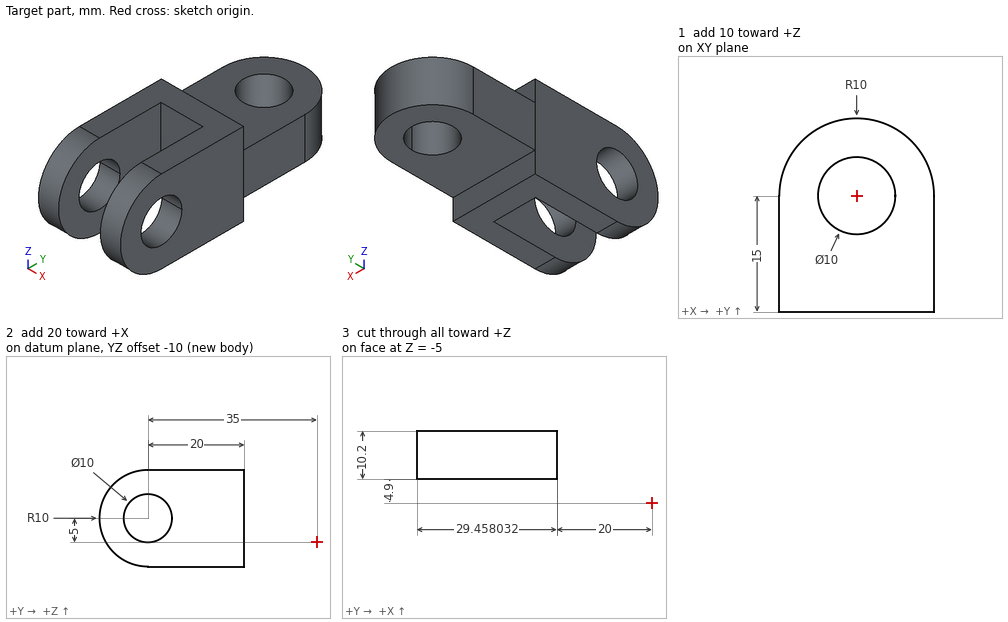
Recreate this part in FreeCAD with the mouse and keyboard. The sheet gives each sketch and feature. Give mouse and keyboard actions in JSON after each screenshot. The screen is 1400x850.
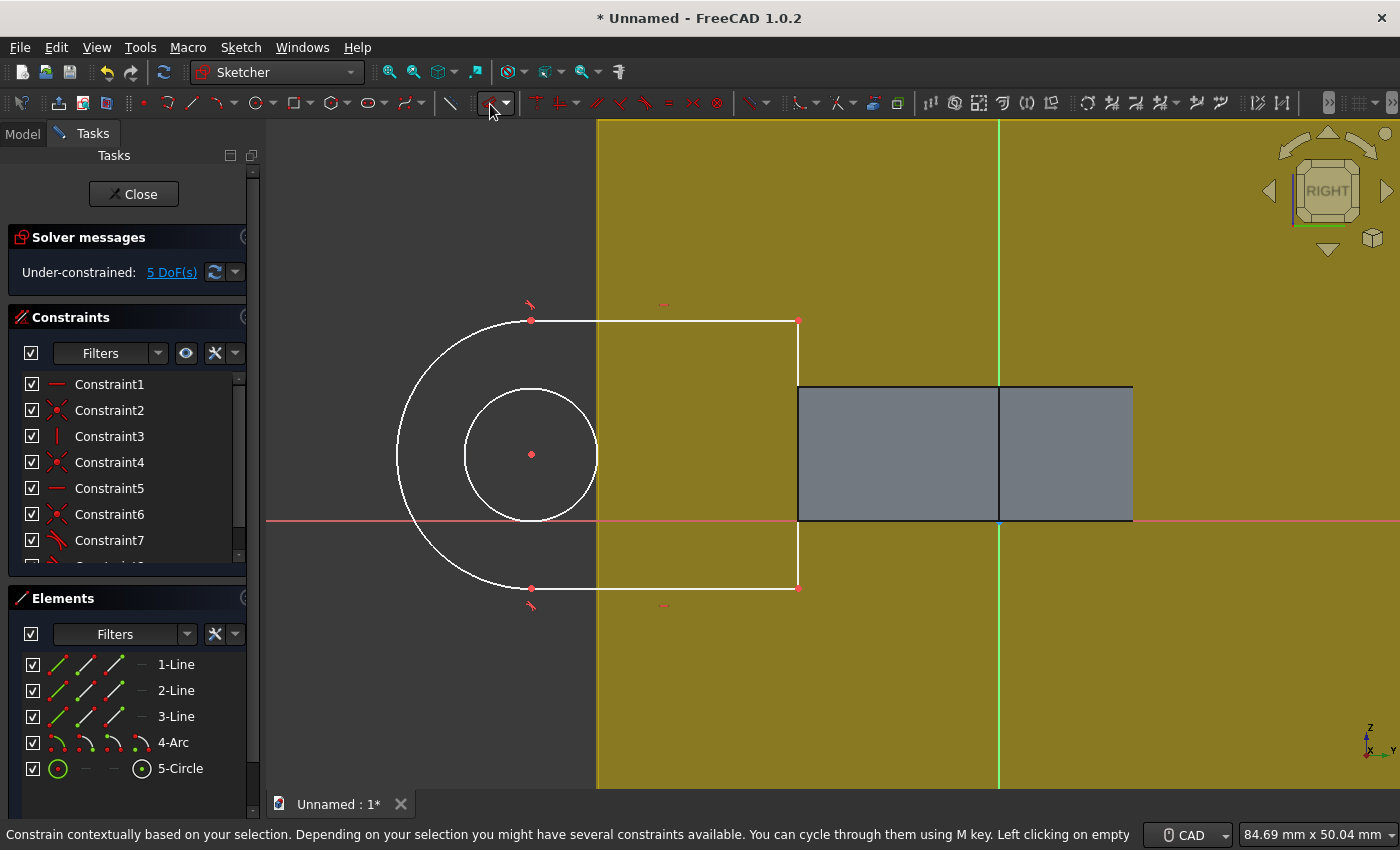
{"action": "left_click", "coordinate": [423, 376]}
{"action": "left_click", "coordinate": [397, 357]}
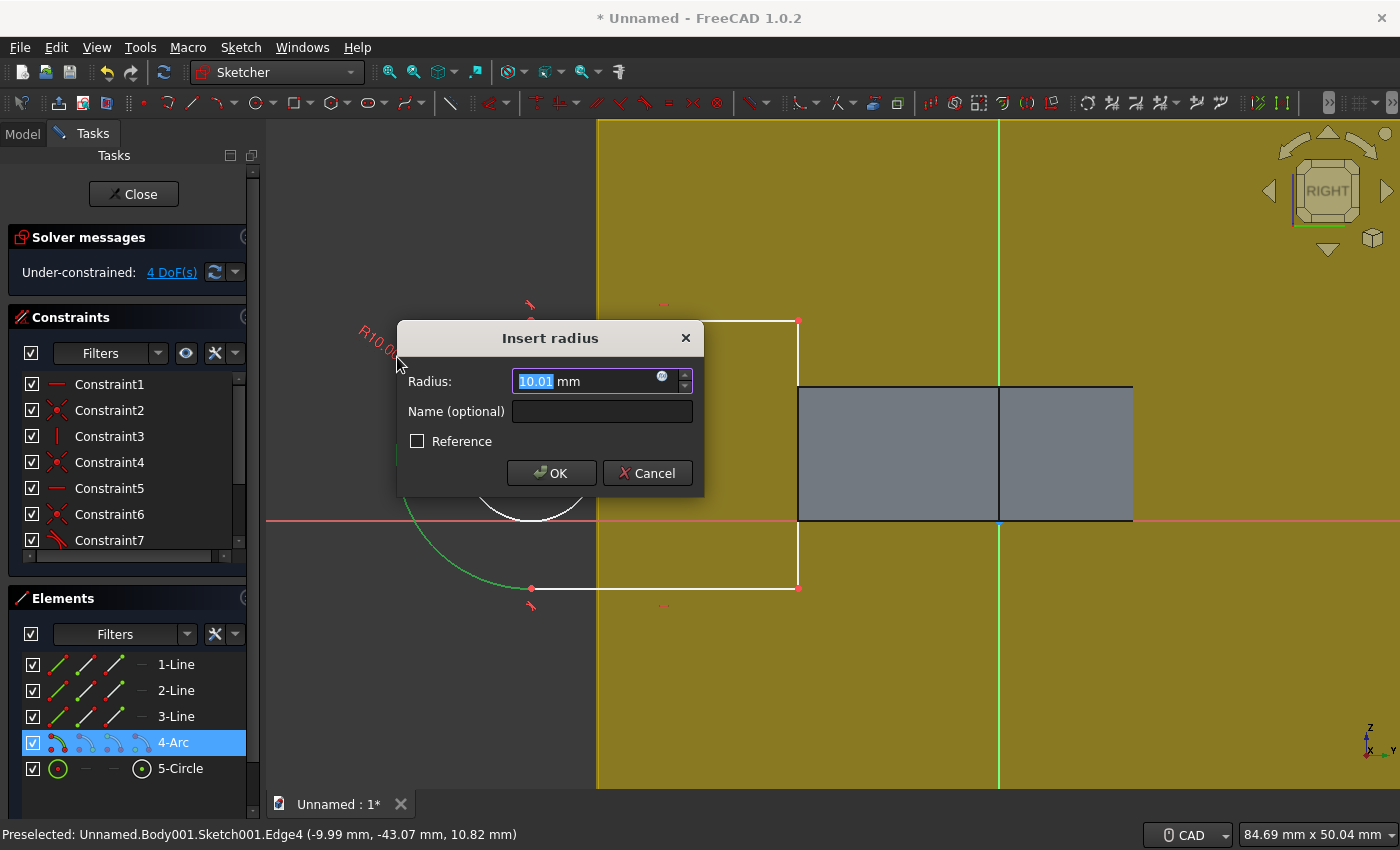
{"action": "type", "text": "10"}
{"action": "key", "text": "Return"}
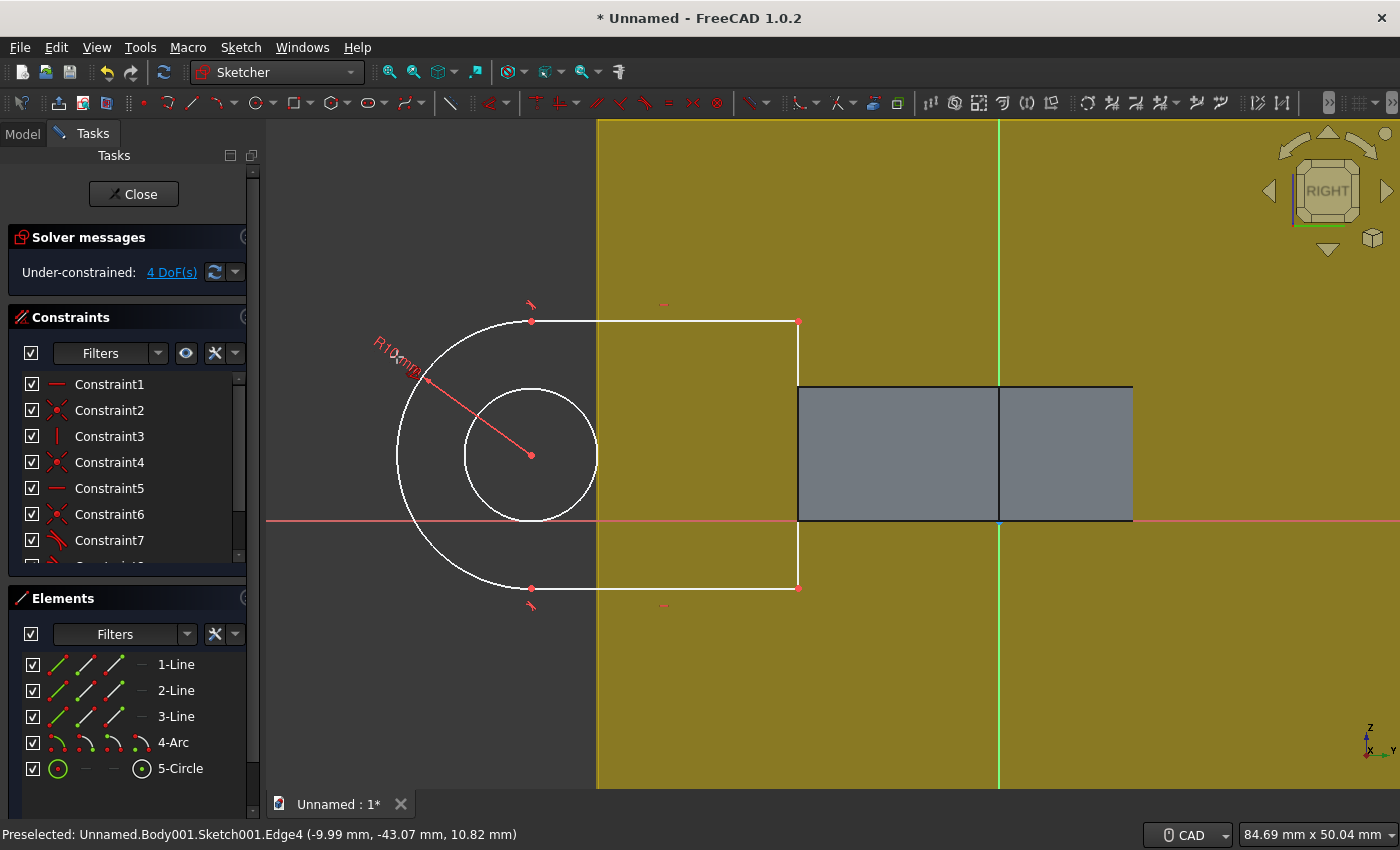
{"action": "left_click", "coordinate": [578, 408]}
{"action": "left_click", "coordinate": [601, 385]}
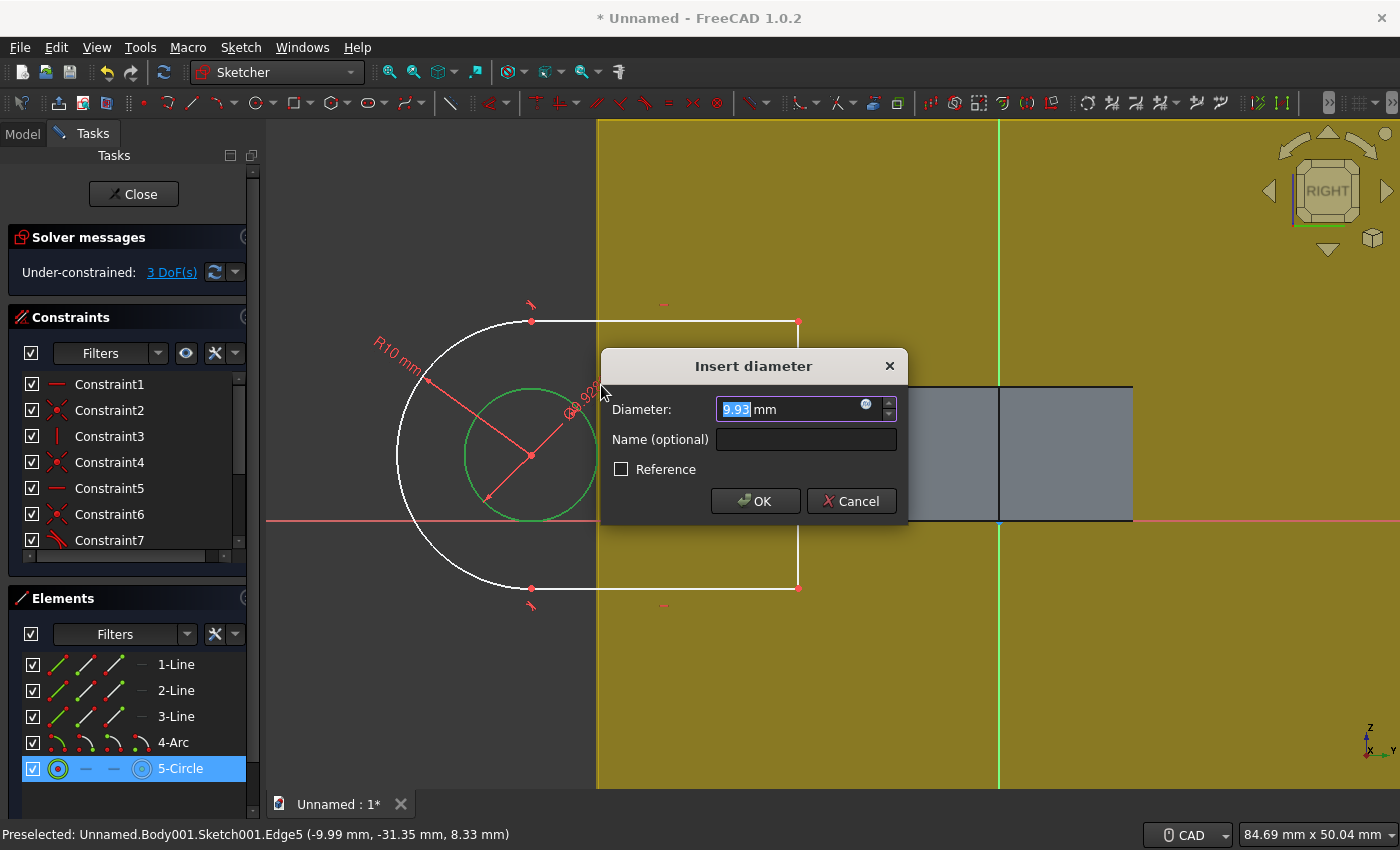
{"action": "type", "text": "10"}
{"action": "key", "text": "Return"}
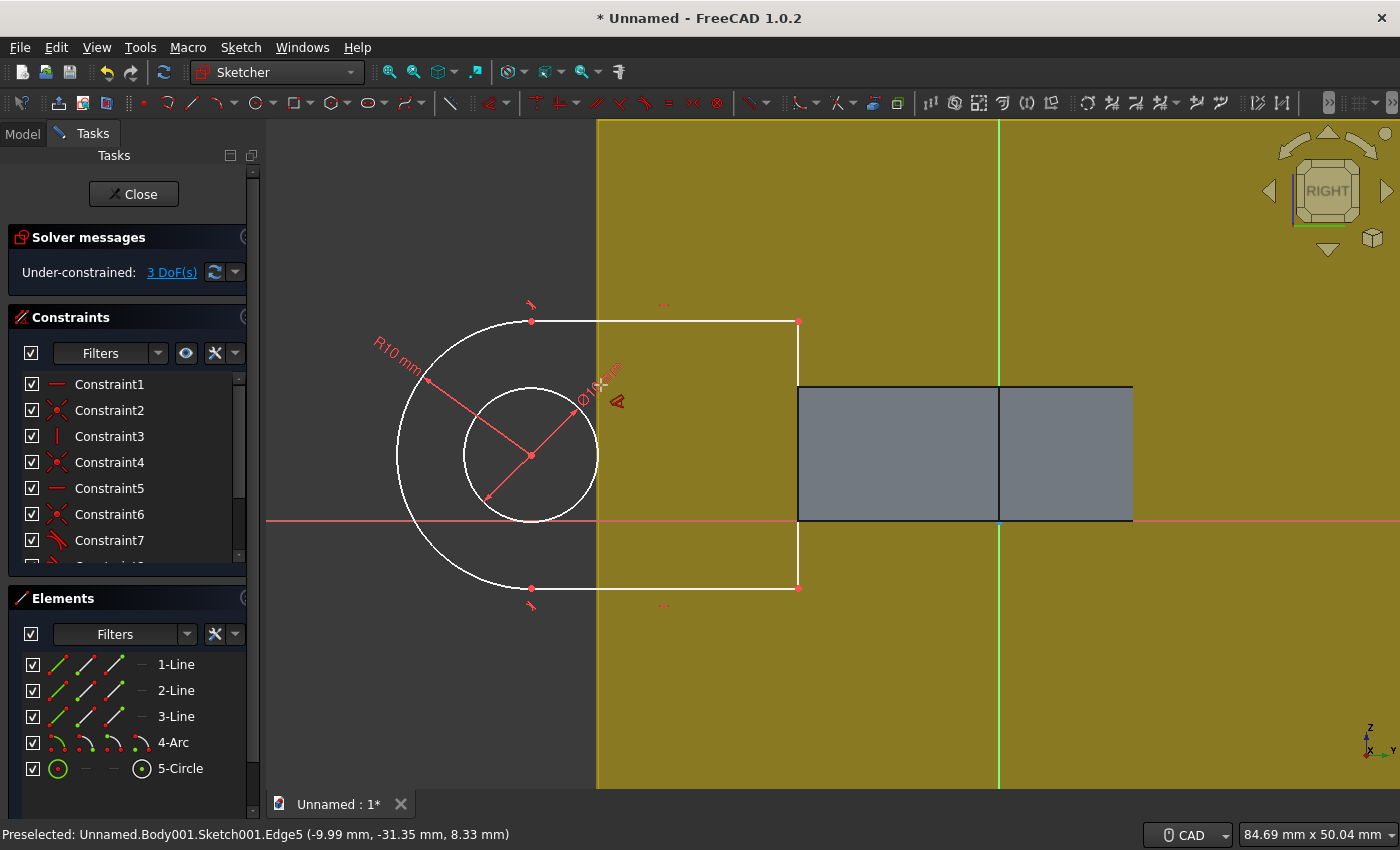
{"action": "left_click", "coordinate": [531, 455]}
{"action": "left_click", "coordinate": [1033, 488]}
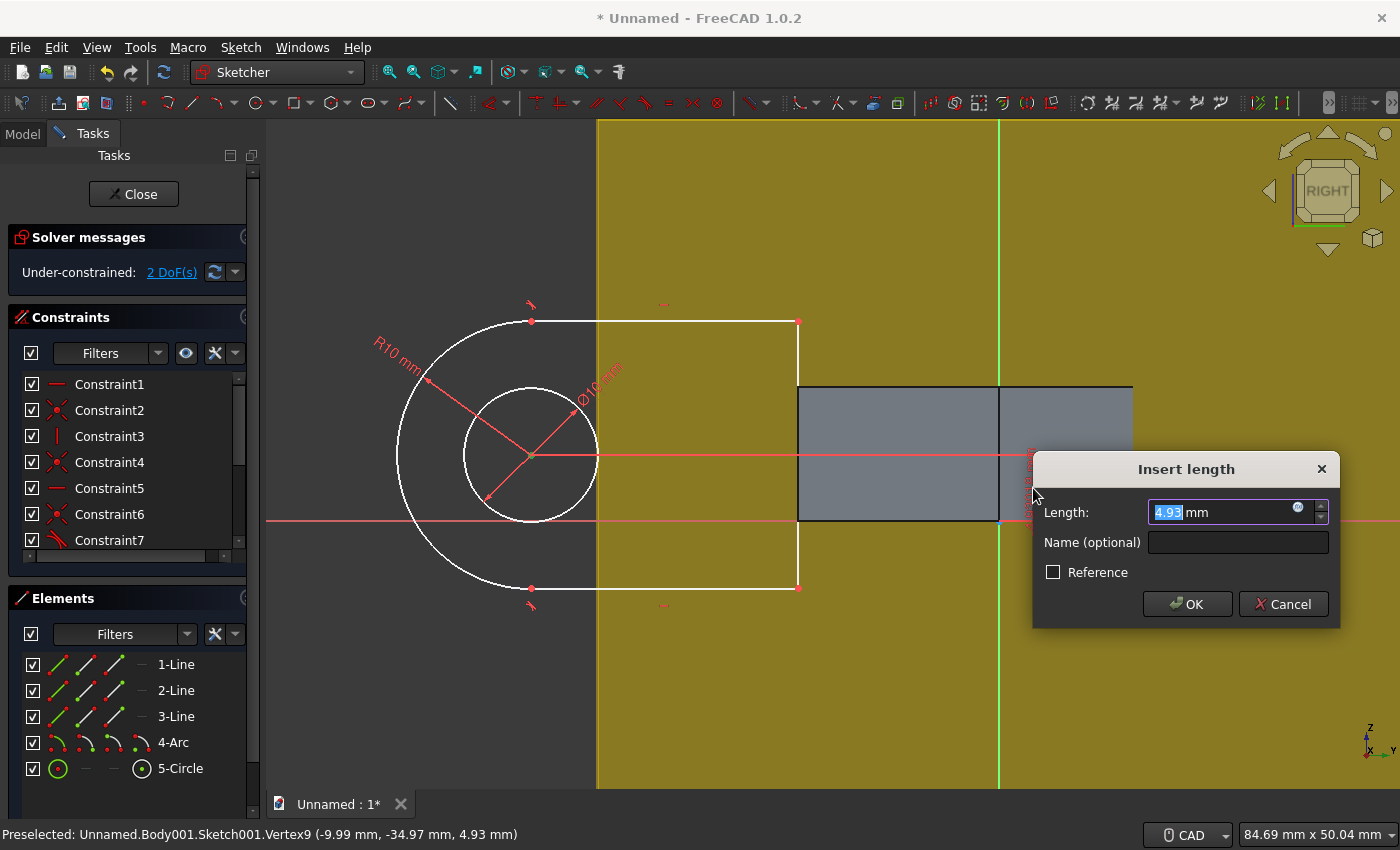
{"action": "type", "text": "5"}
{"action": "key", "text": "Return"}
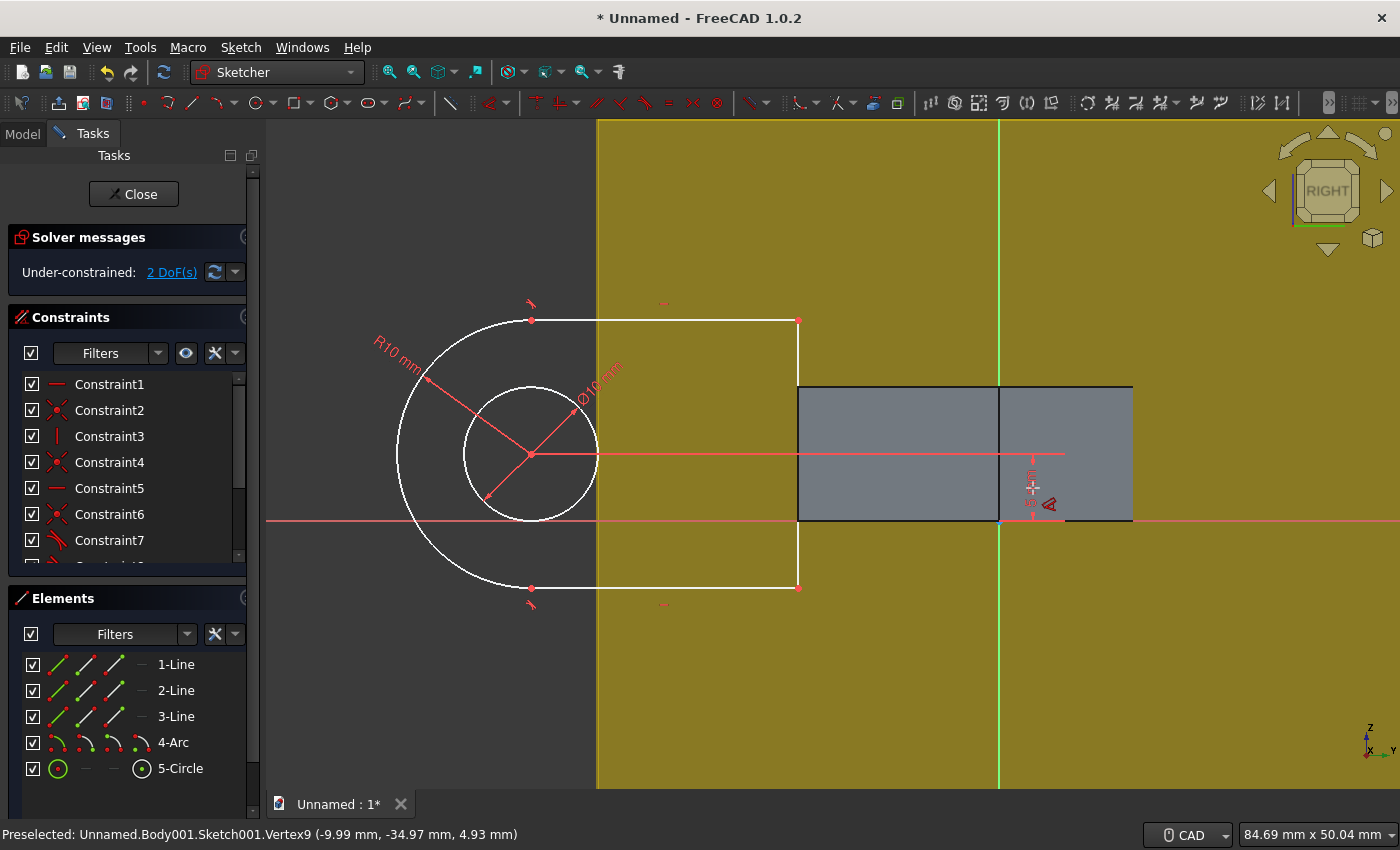
{"action": "left_click", "coordinate": [611, 320]}
{"action": "left_click", "coordinate": [665, 286]}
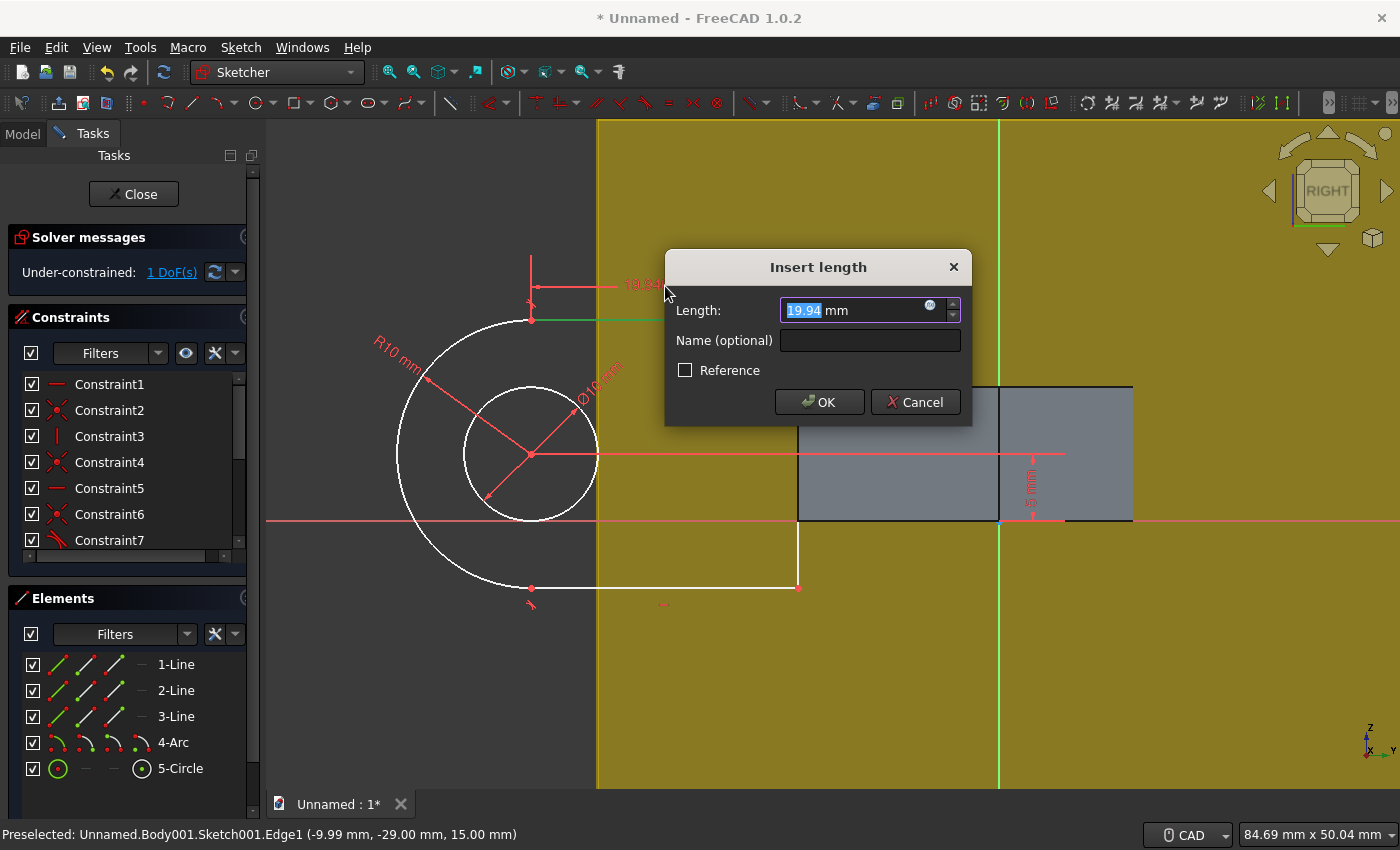
{"action": "type", "text": "20"}
{"action": "key", "text": "Return"}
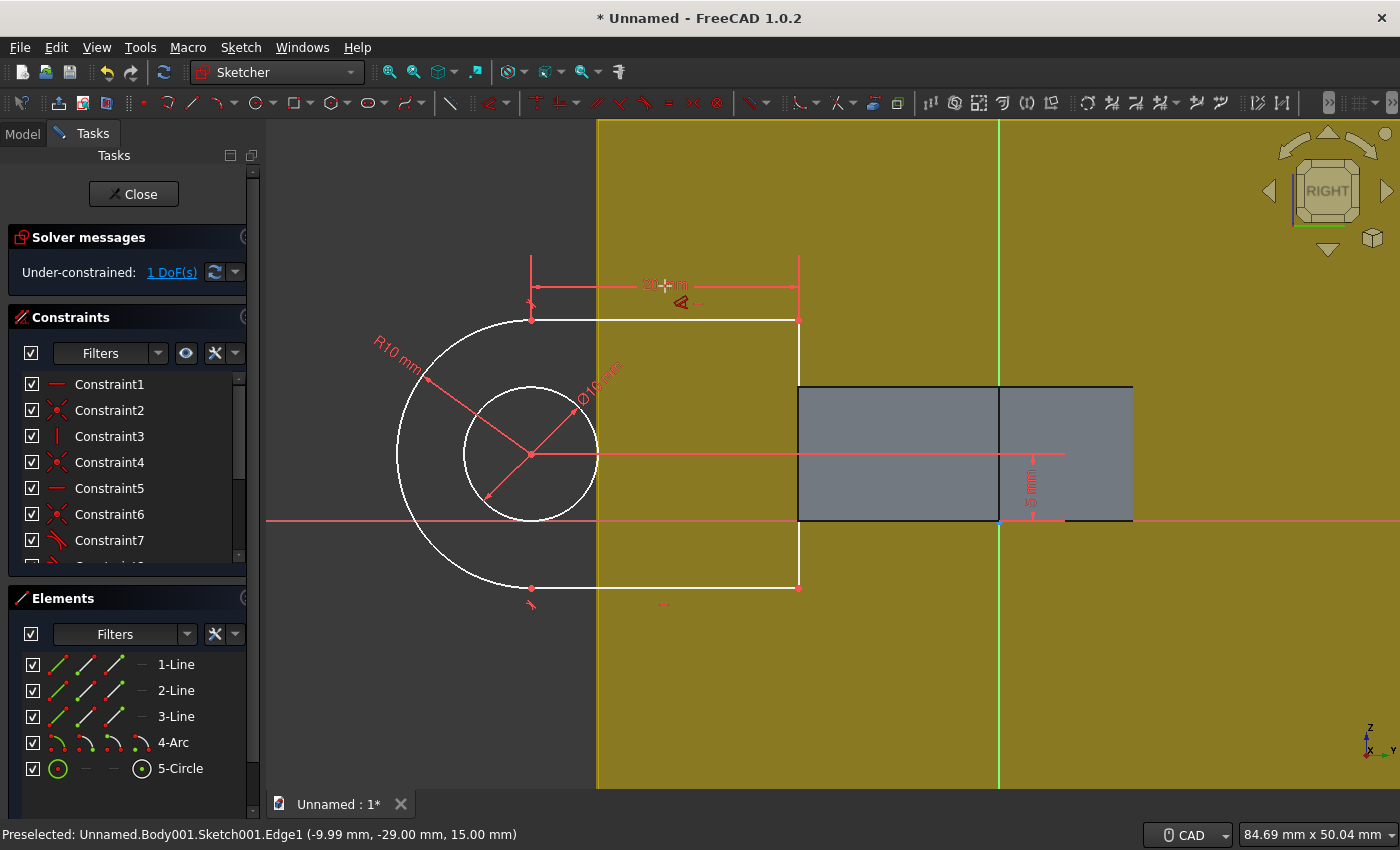
{"action": "left_click", "coordinate": [531, 454]}
{"action": "left_click", "coordinate": [765, 555]}